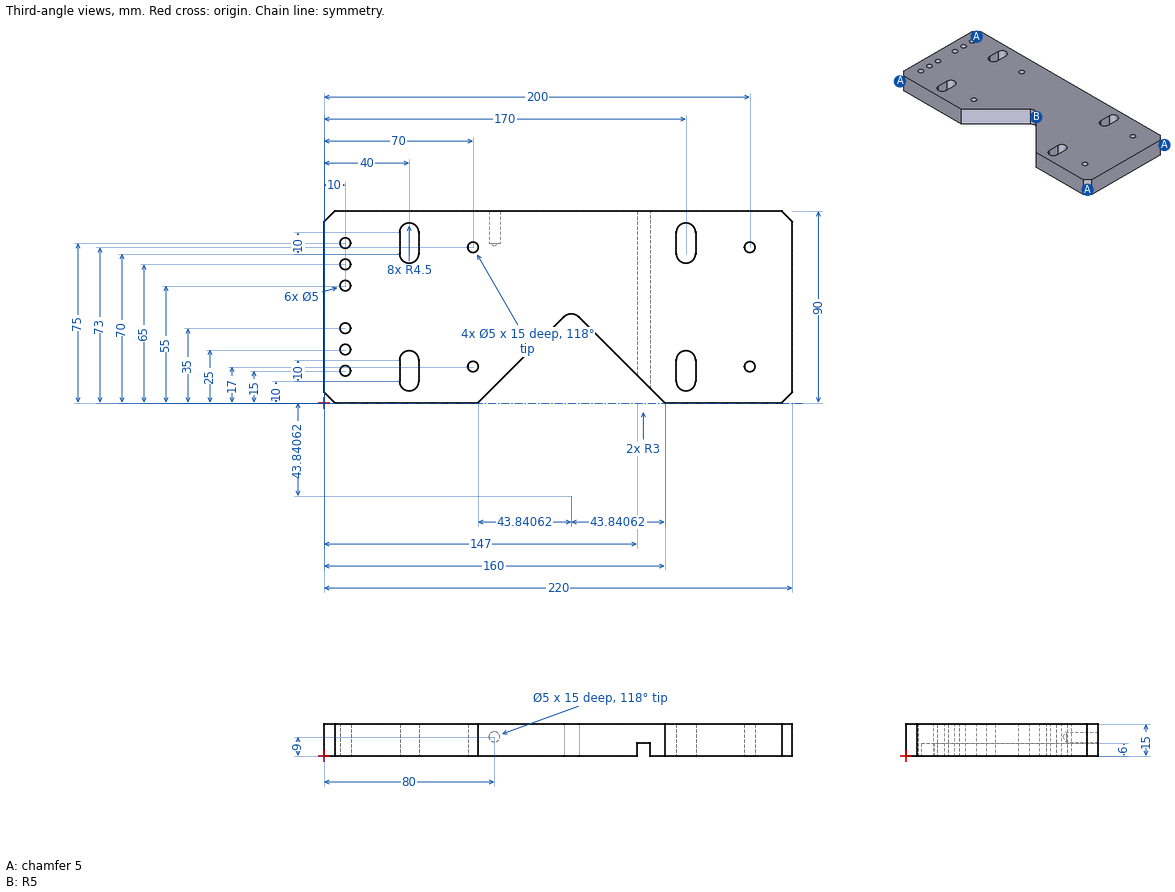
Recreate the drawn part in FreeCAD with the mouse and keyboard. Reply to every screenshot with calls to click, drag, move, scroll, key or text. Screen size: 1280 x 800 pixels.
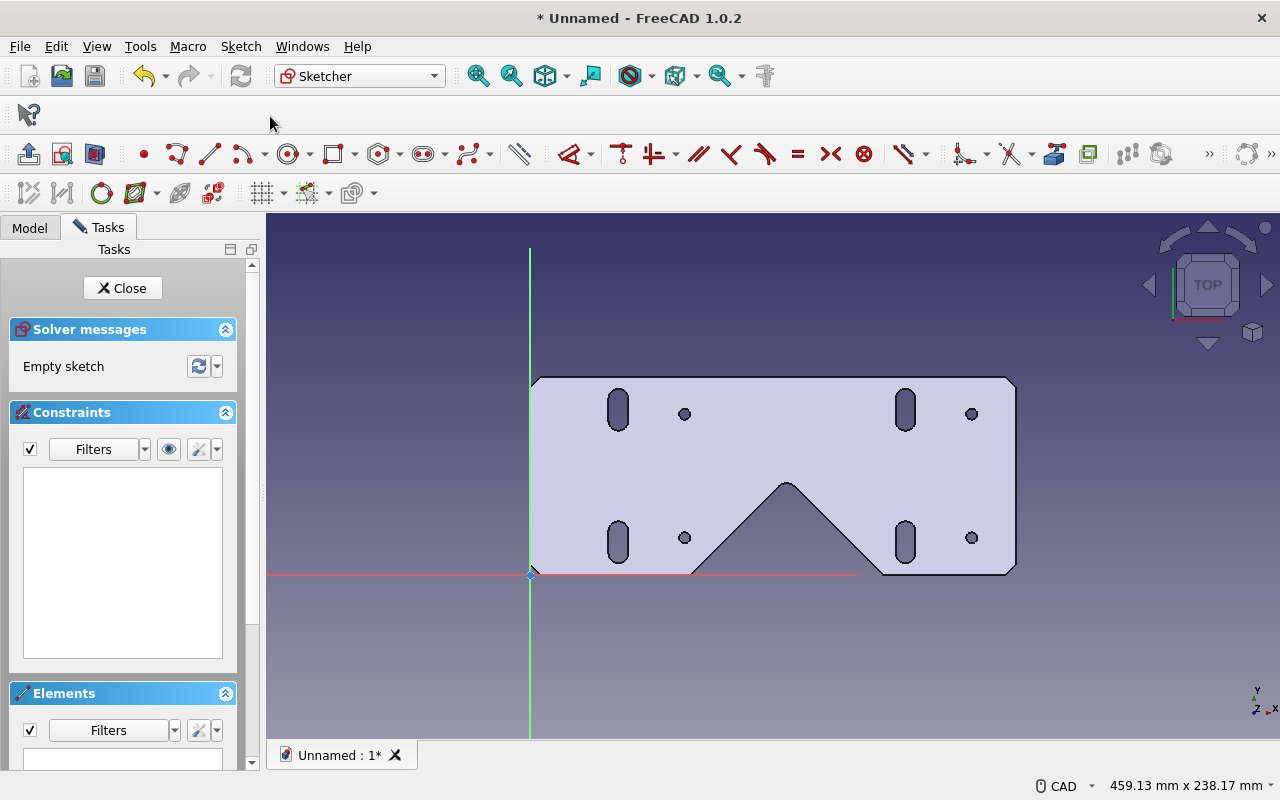
scroll(348, 507, up, 3)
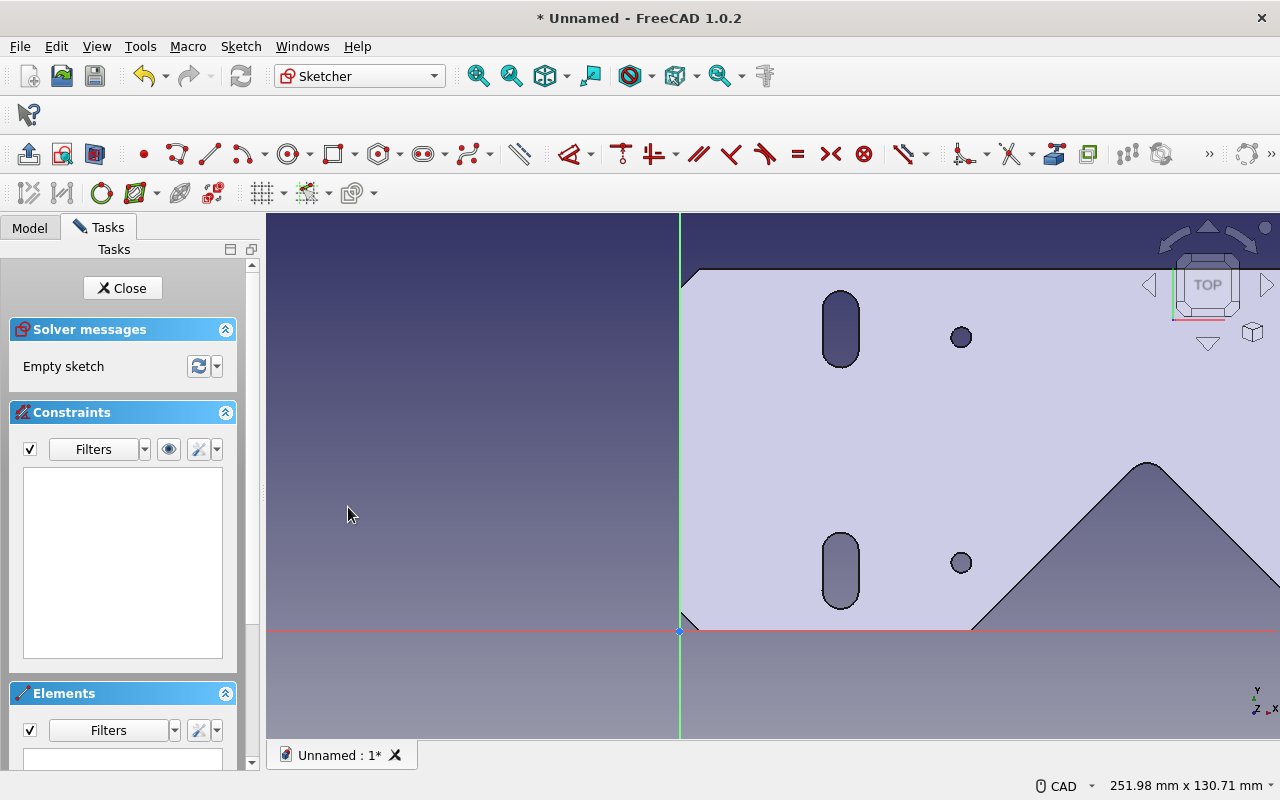
click(288, 154)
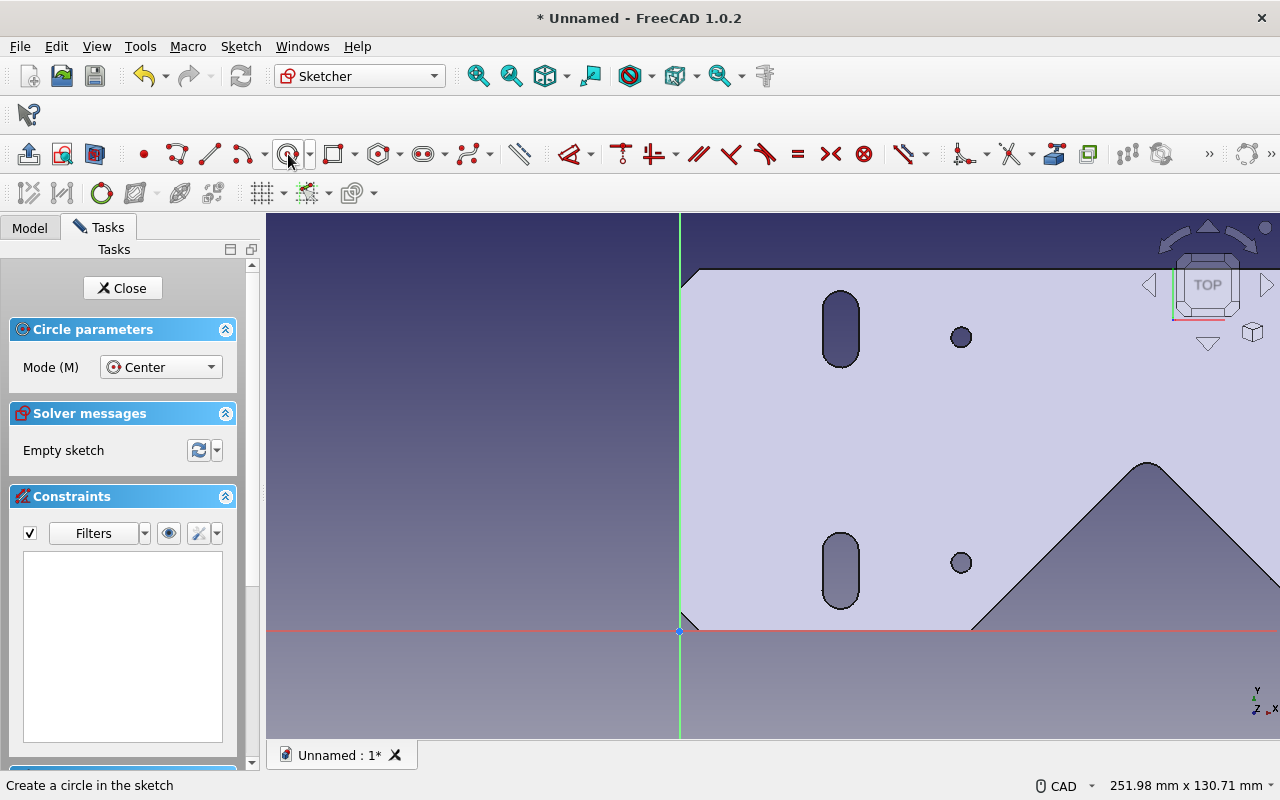
scroll(720, 410, up, 5)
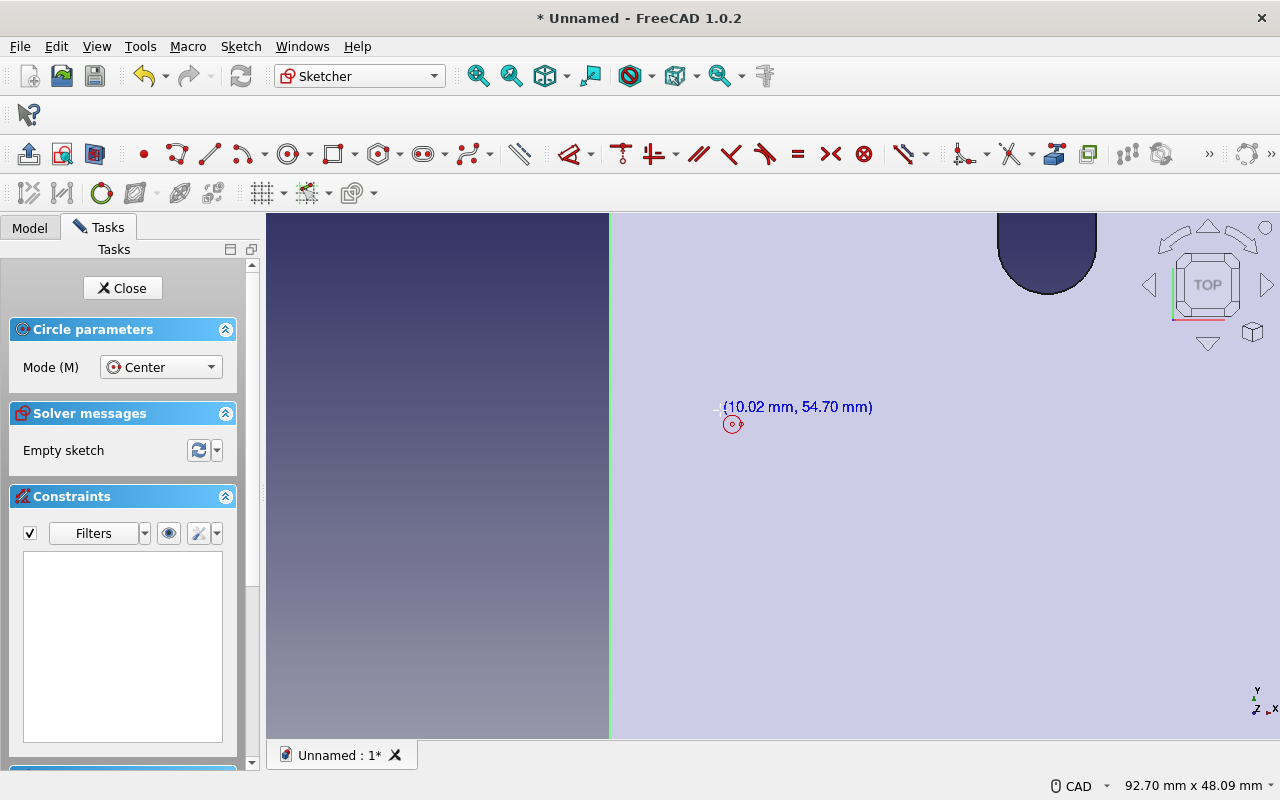
click(719, 409)
click(738, 390)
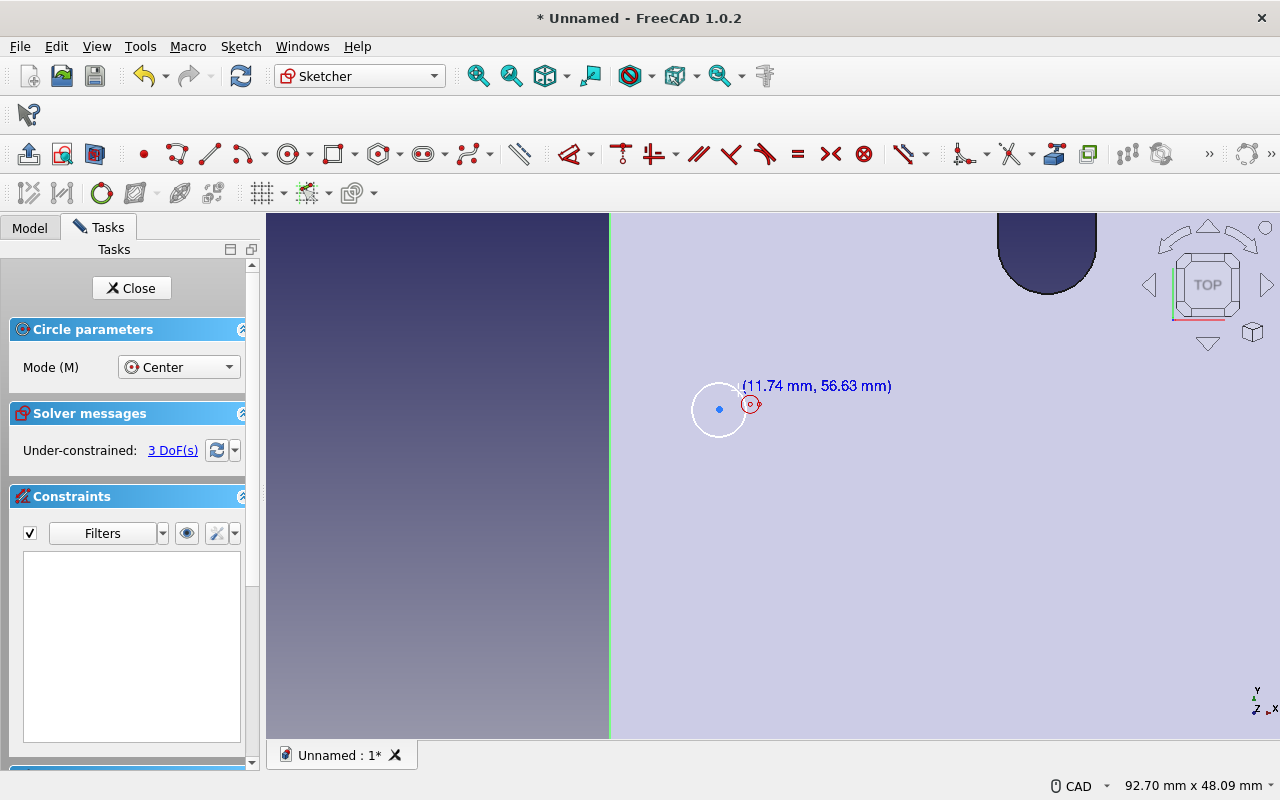
click(719, 628)
click(738, 608)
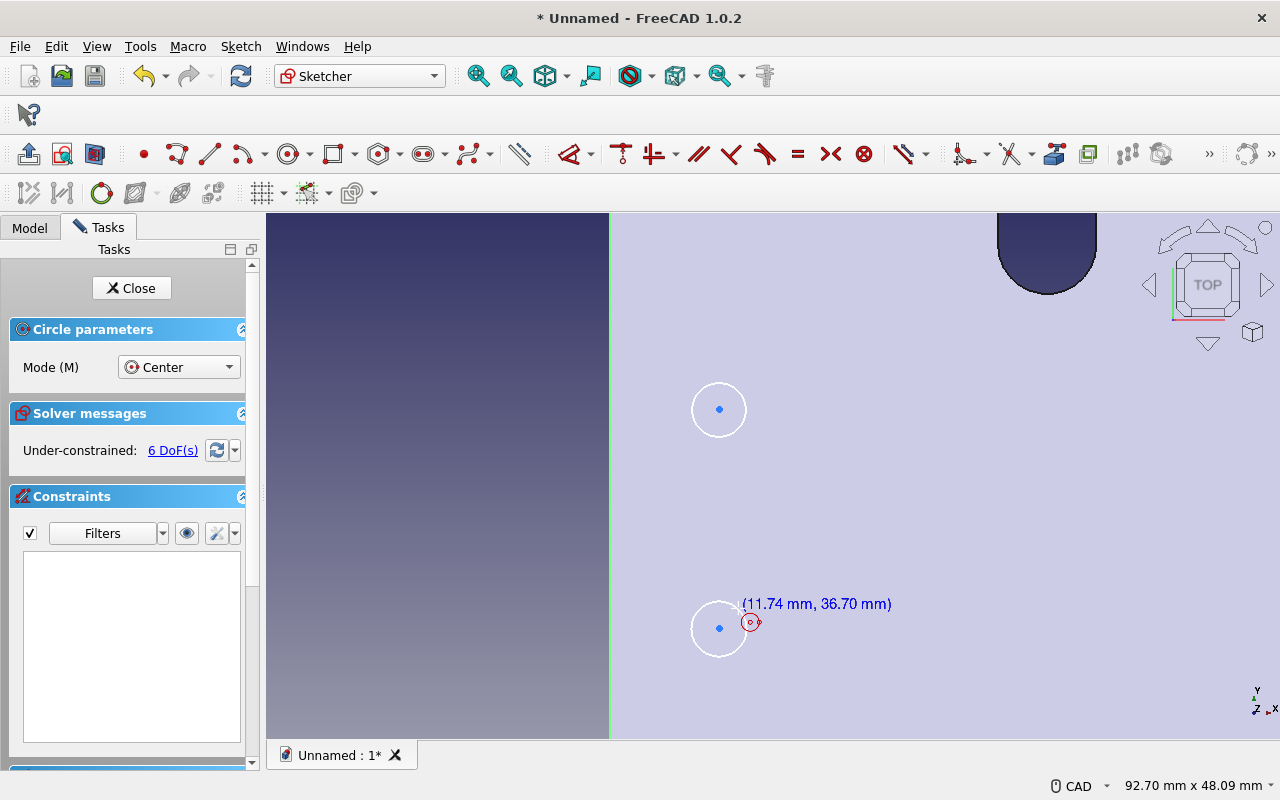
scroll(720, 412, down, 5)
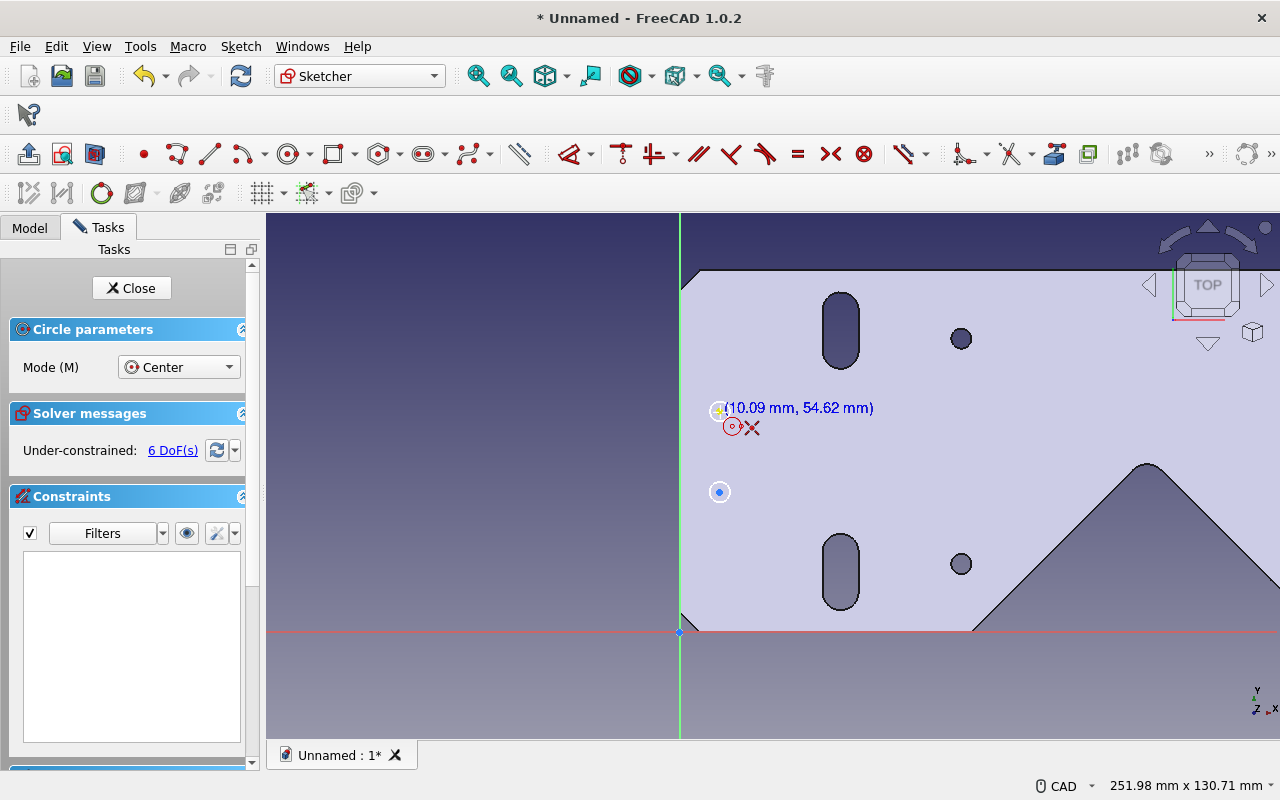
scroll(720, 532, up, 5)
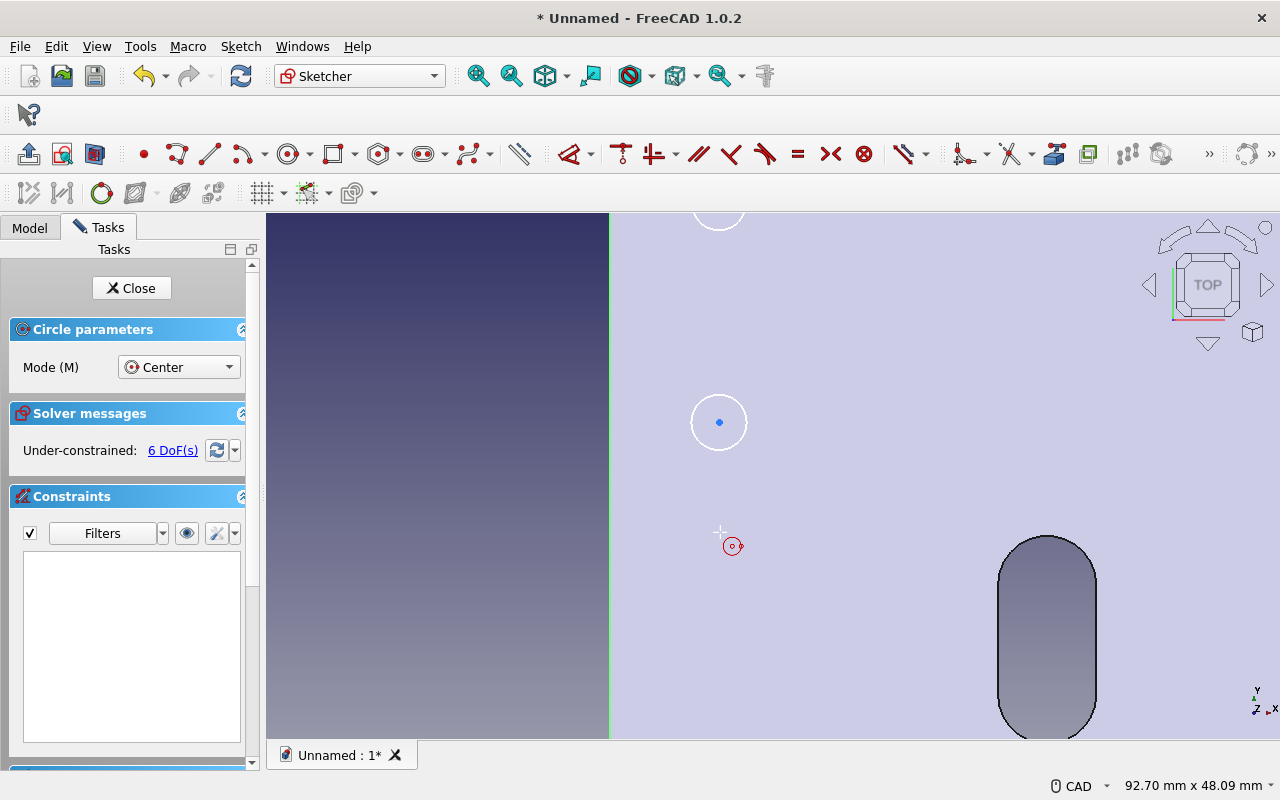
click(719, 530)
click(738, 511)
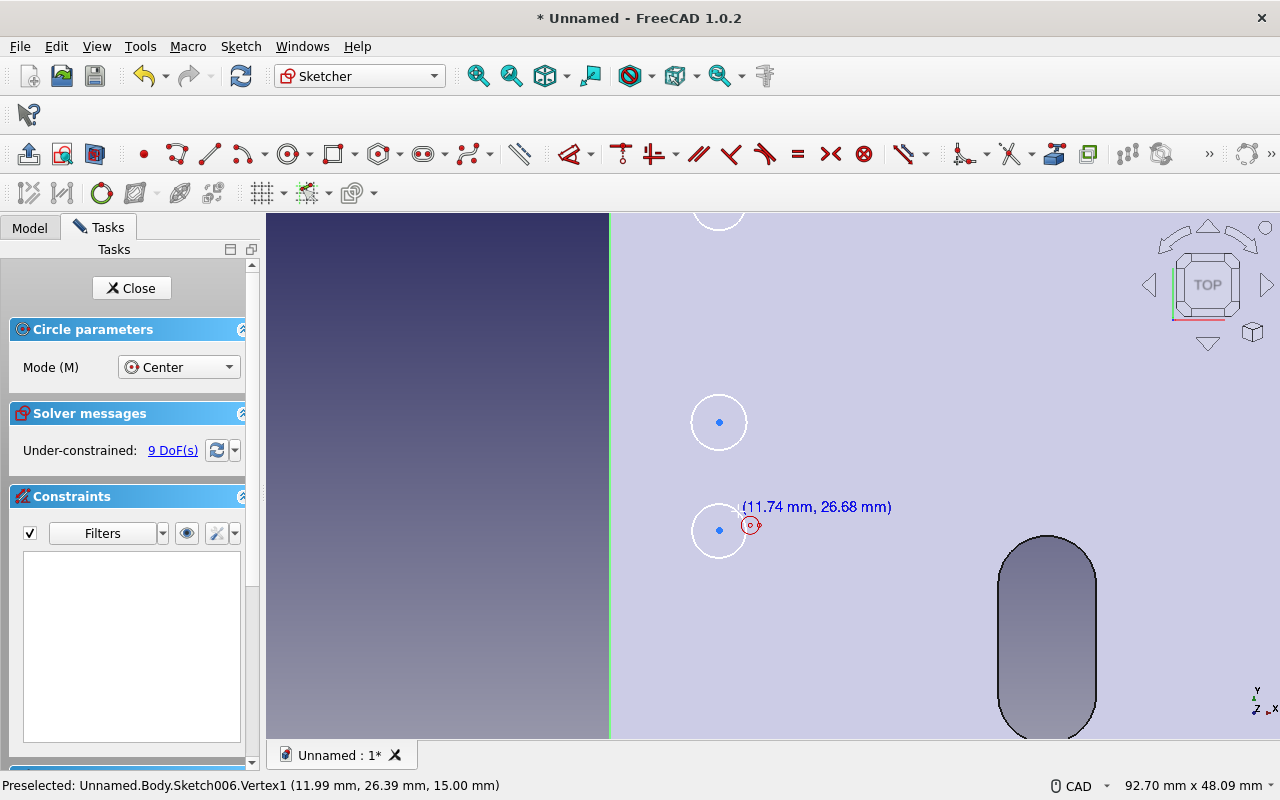
scroll(720, 532, down, 5)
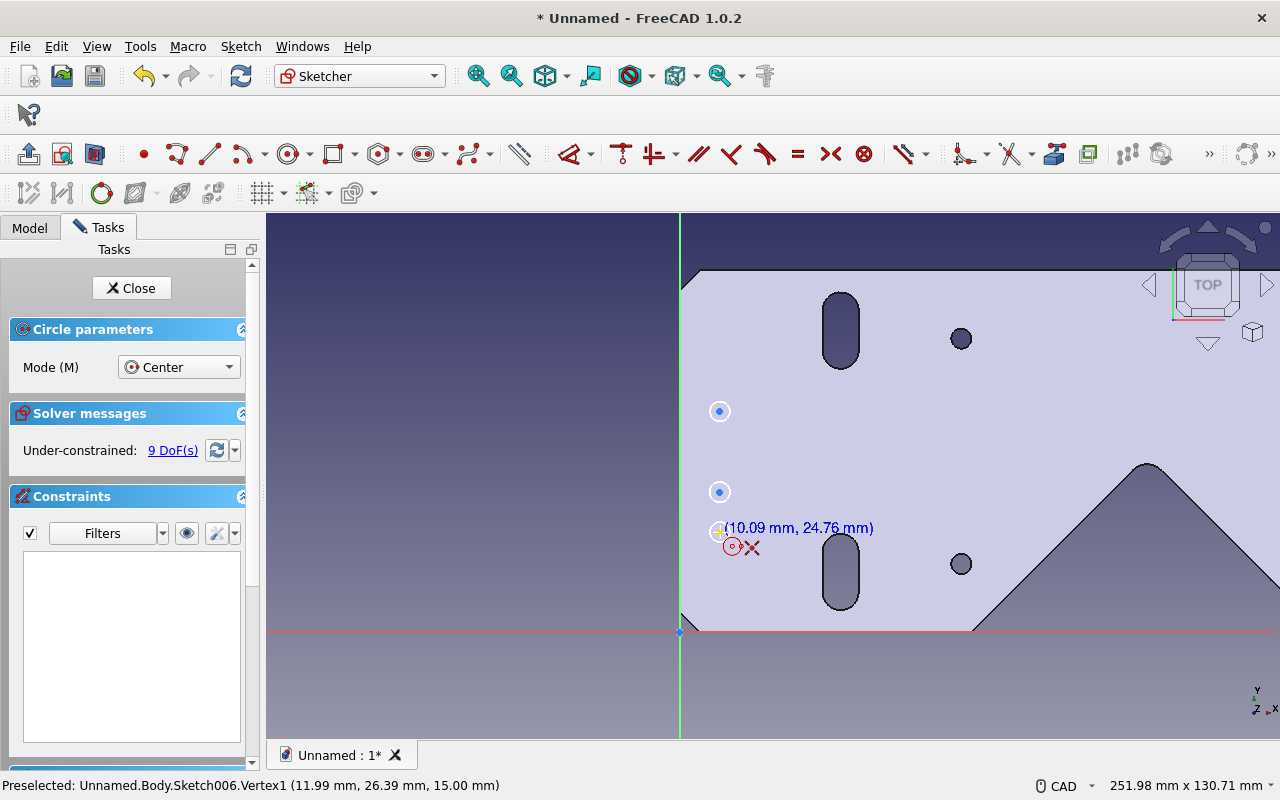
scroll(720, 371, up, 5)